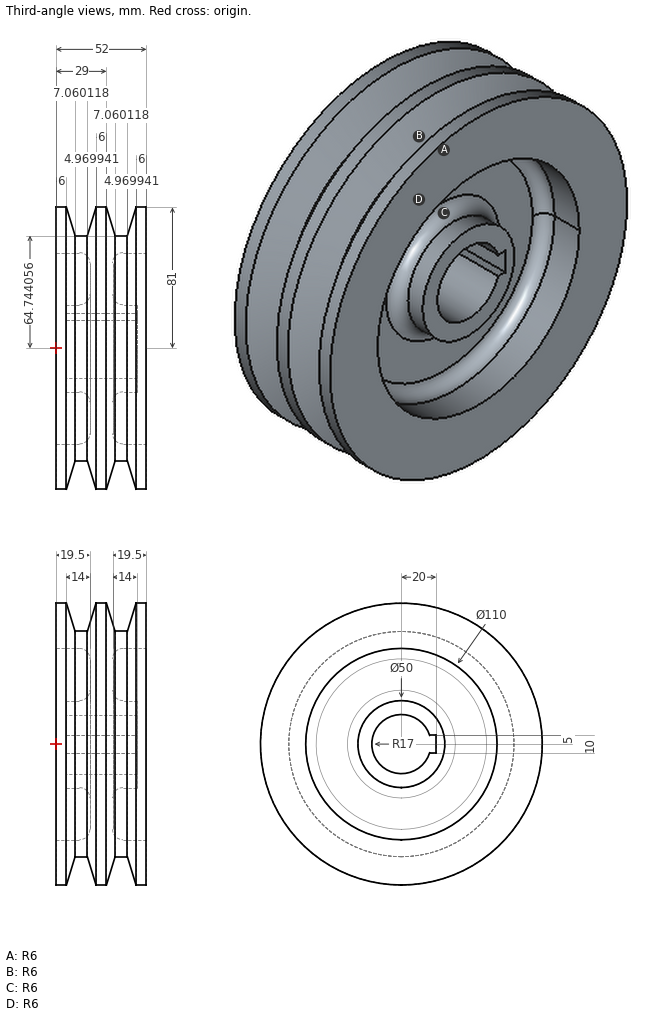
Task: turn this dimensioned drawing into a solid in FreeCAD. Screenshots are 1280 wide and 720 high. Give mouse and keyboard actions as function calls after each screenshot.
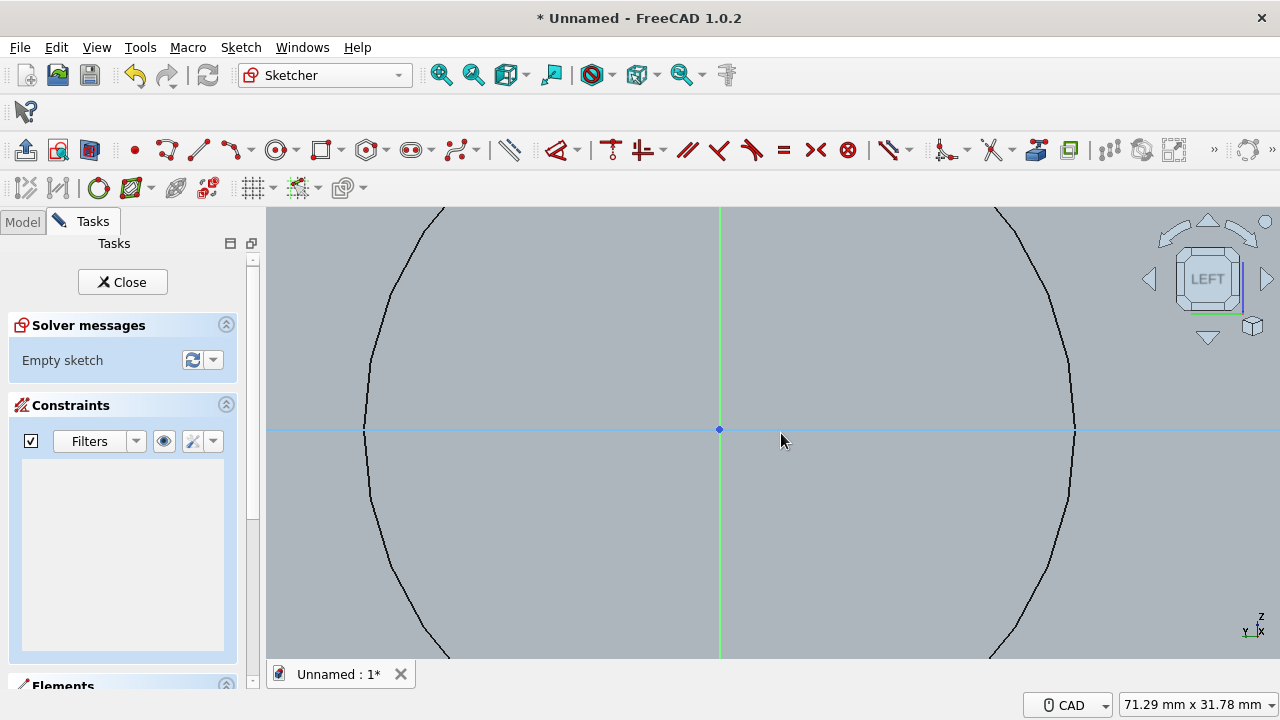
key(g)
key(m)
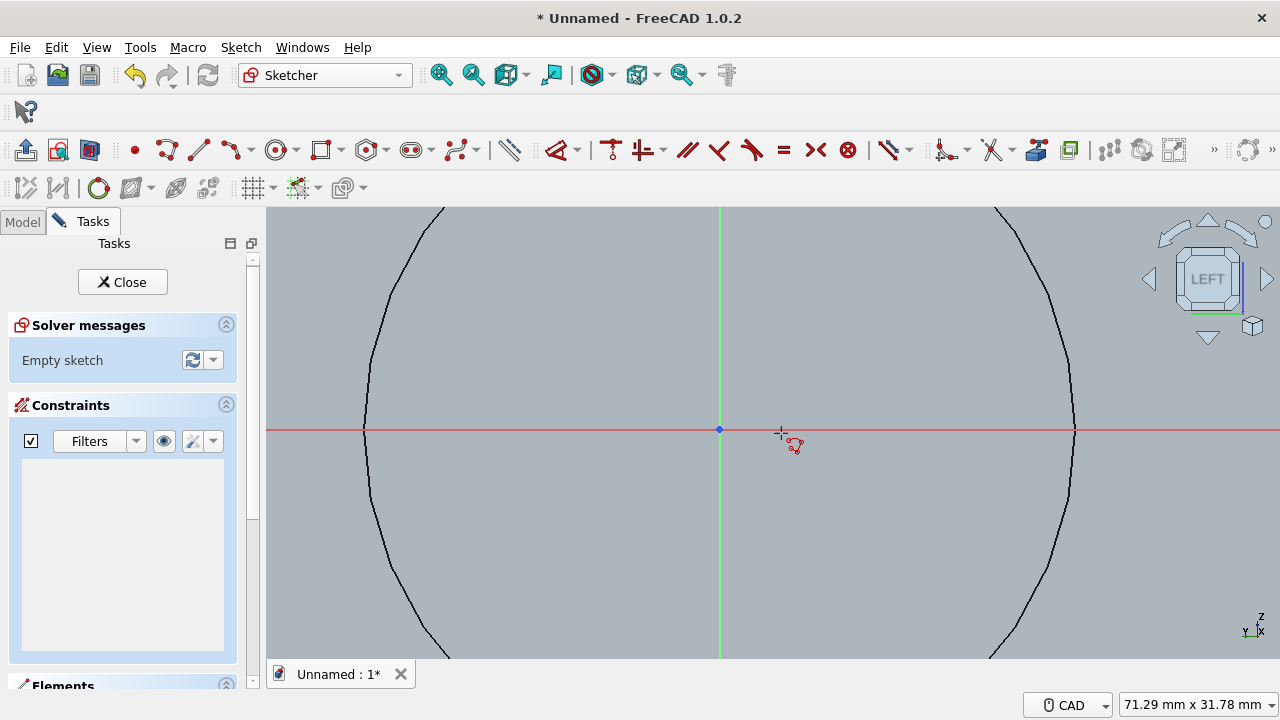
click(488, 359)
click(435, 359)
click(435, 501)
click(488, 501)
right_click(488, 501)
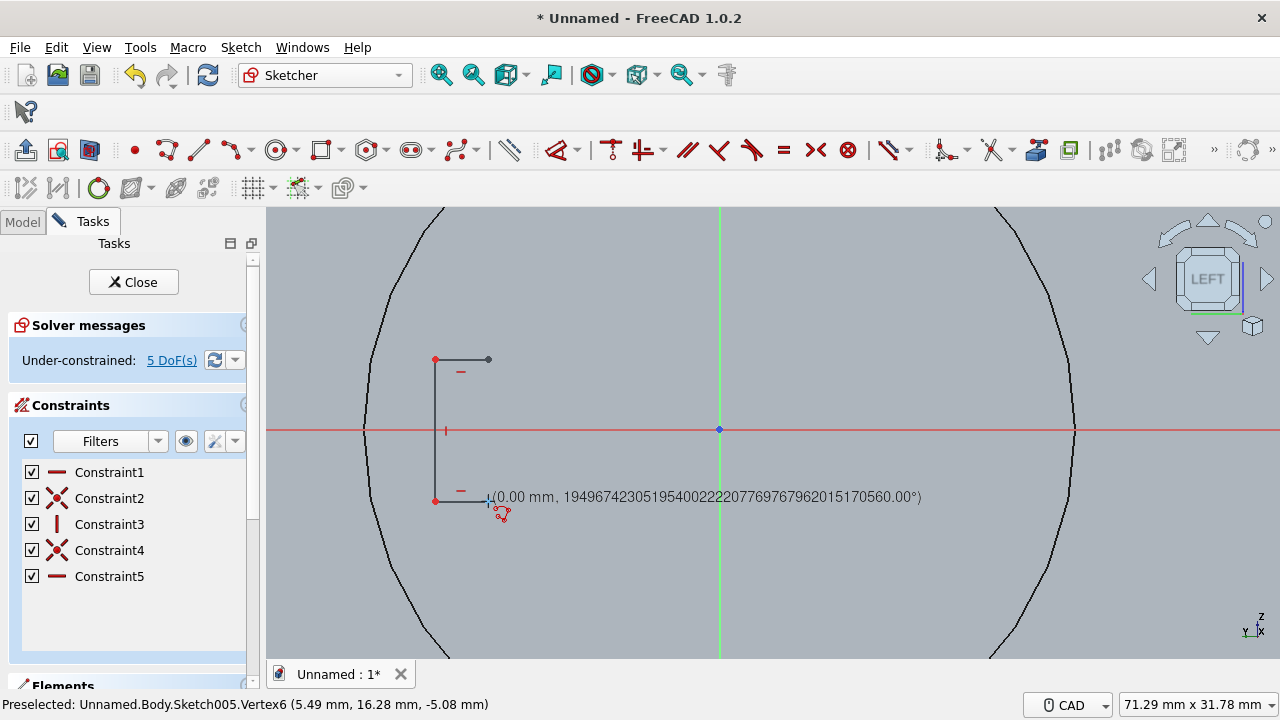
key(g)
key(3)
key(a)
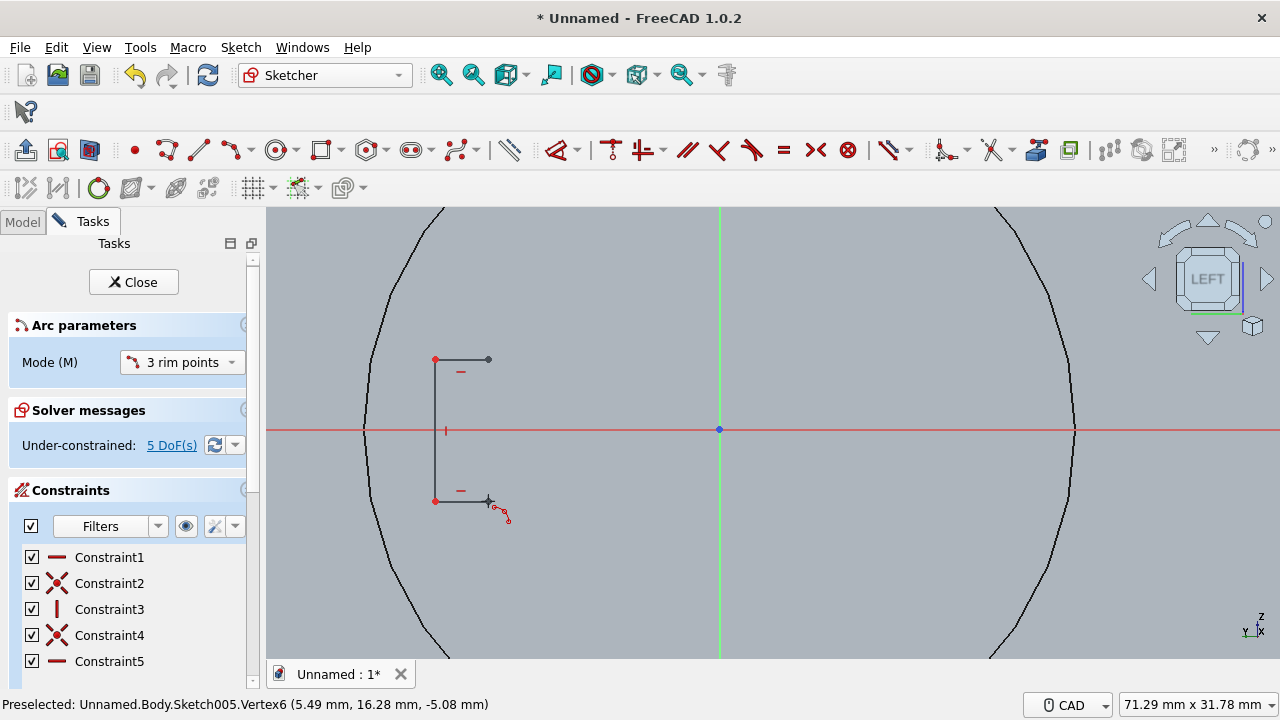
click(488, 502)
click(488, 360)
click(923, 560)
key(Escape)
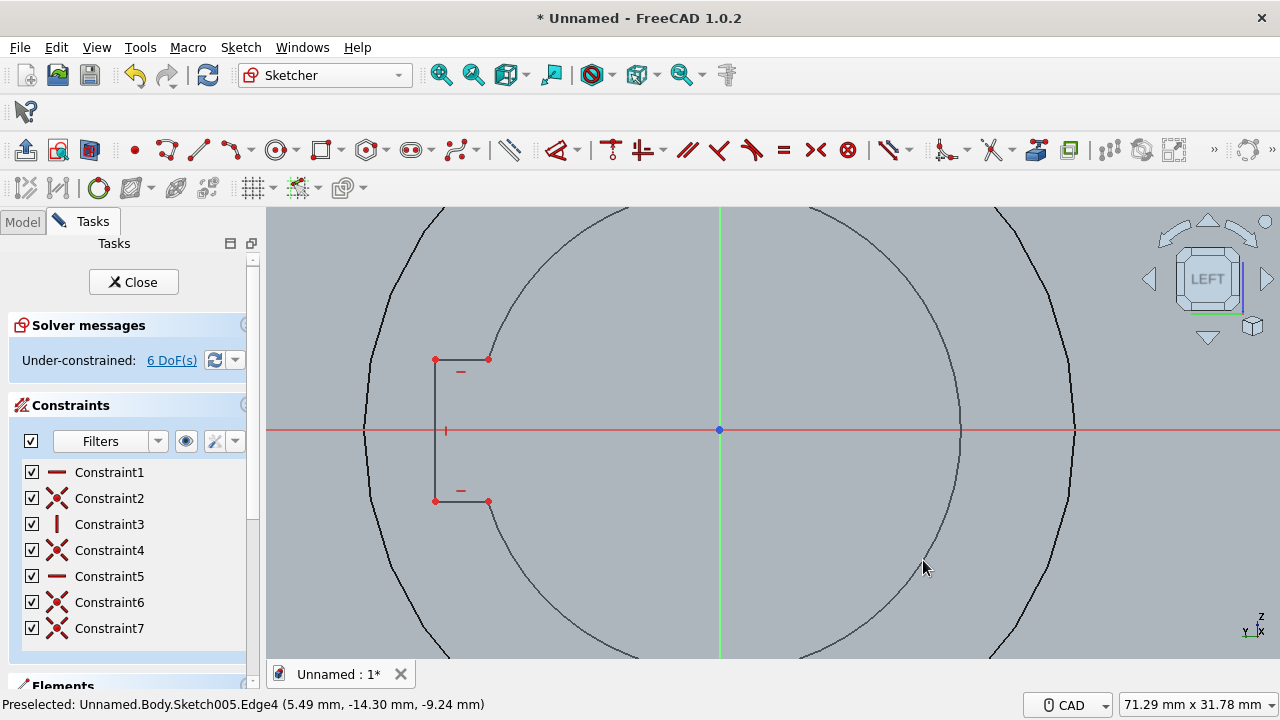
drag(709, 420, 730, 441)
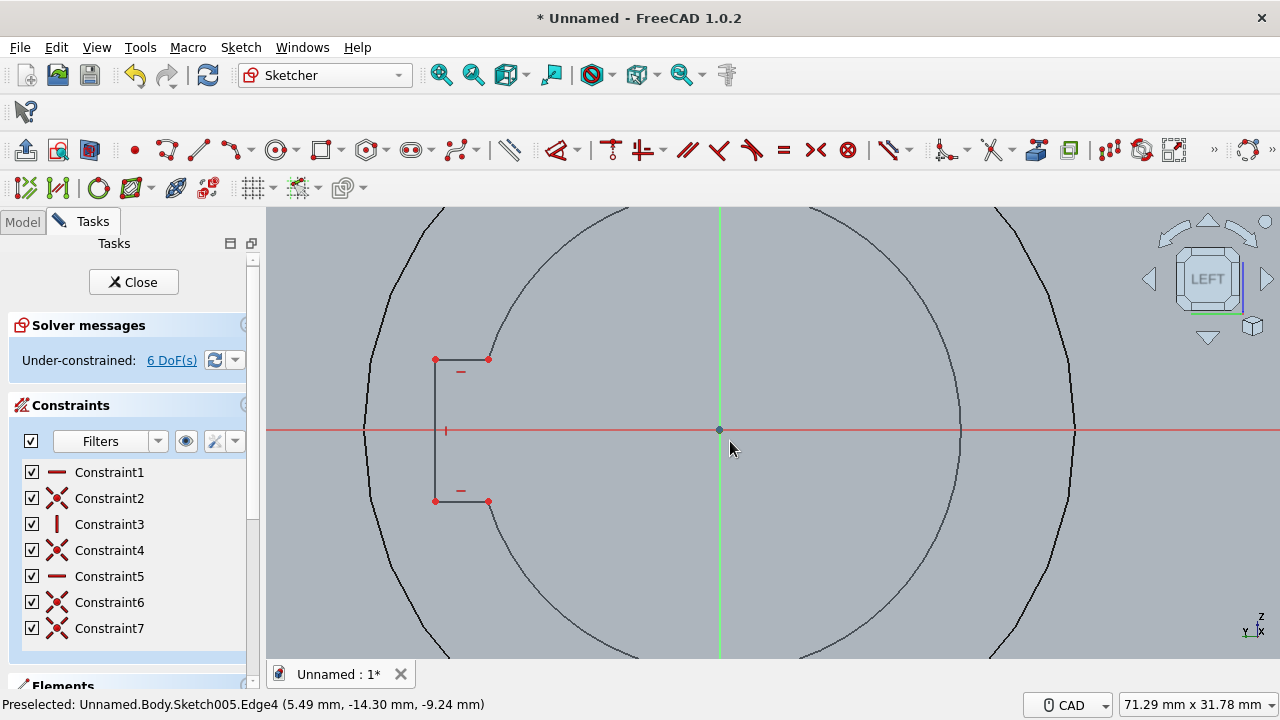
key(c)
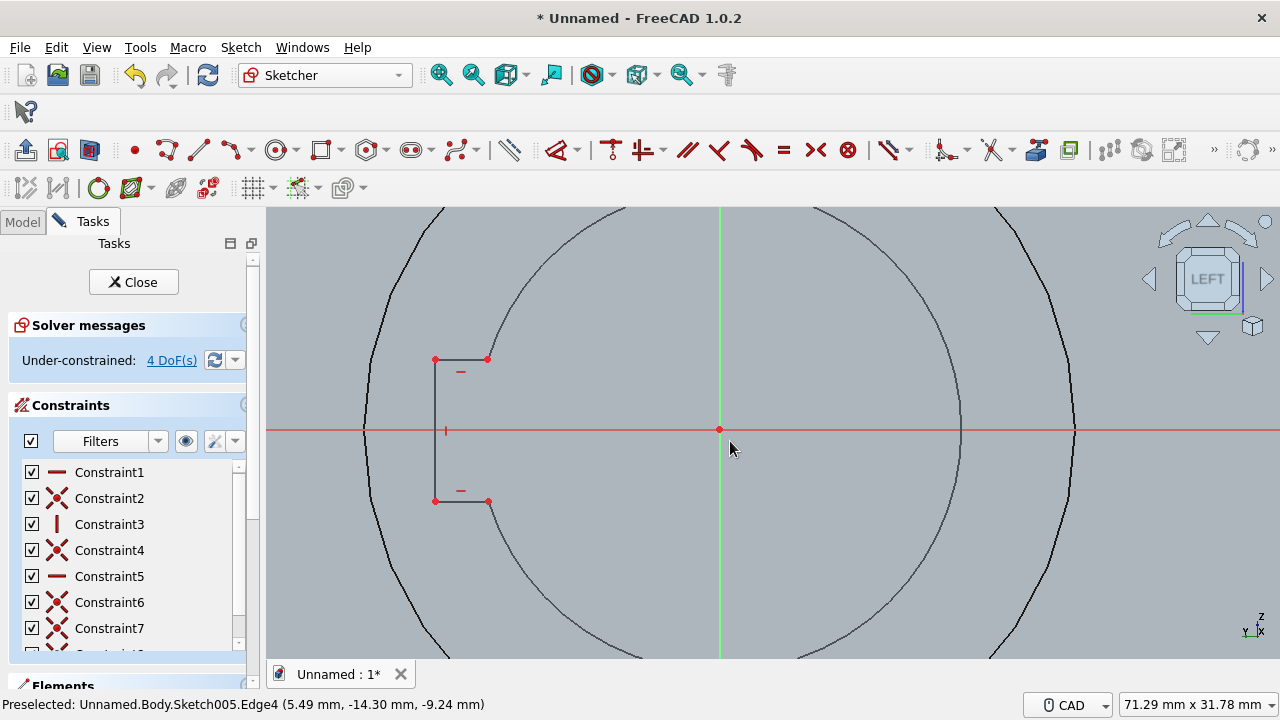
key(d)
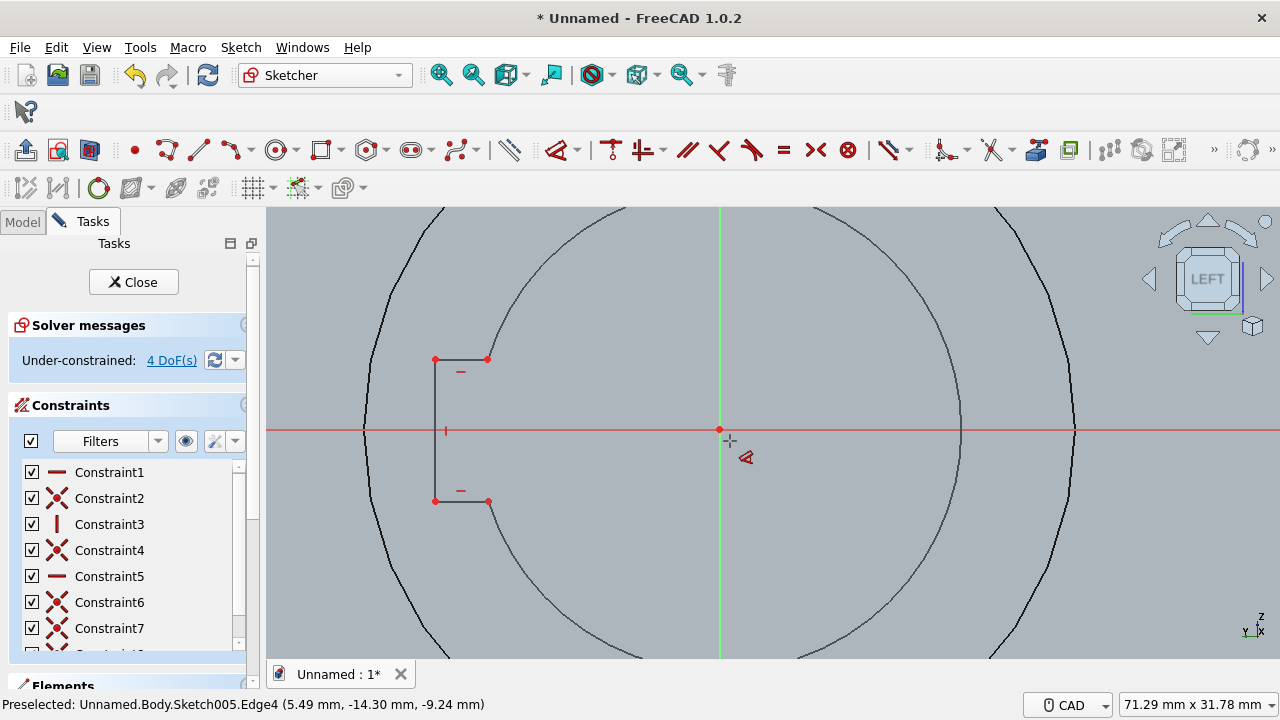
click(961, 429)
click(960, 560)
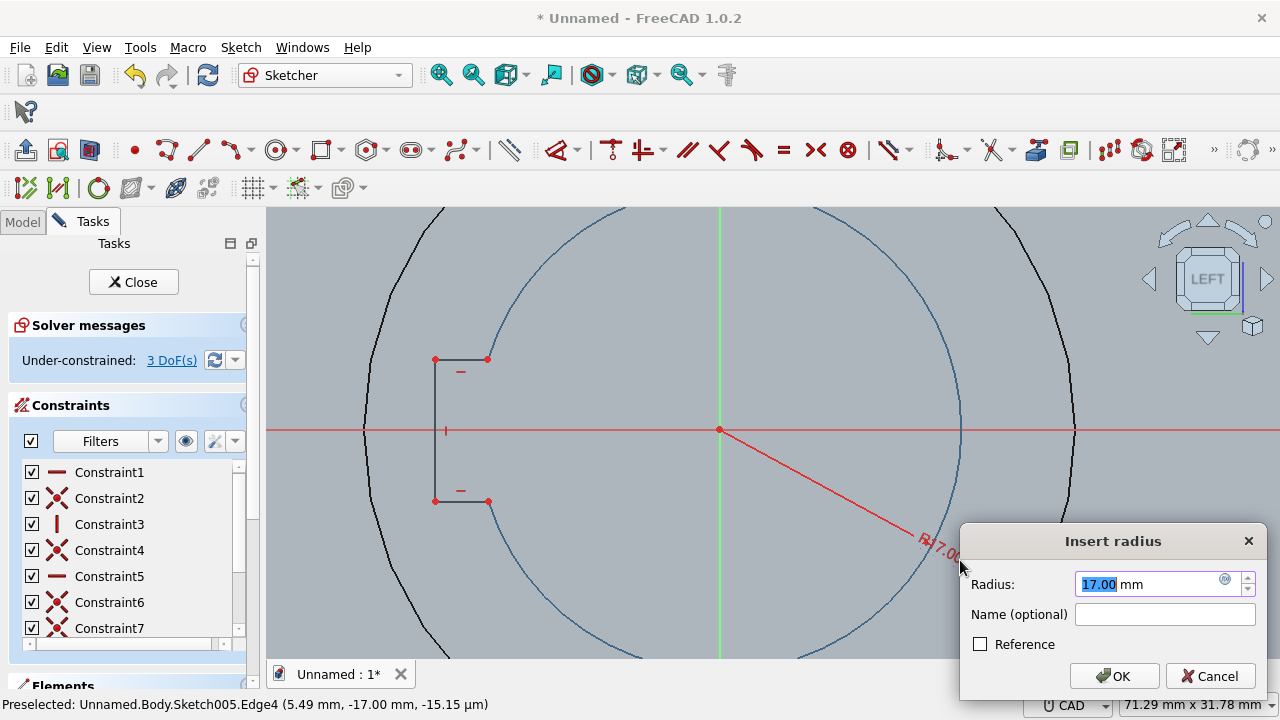
text(17)
key(Return)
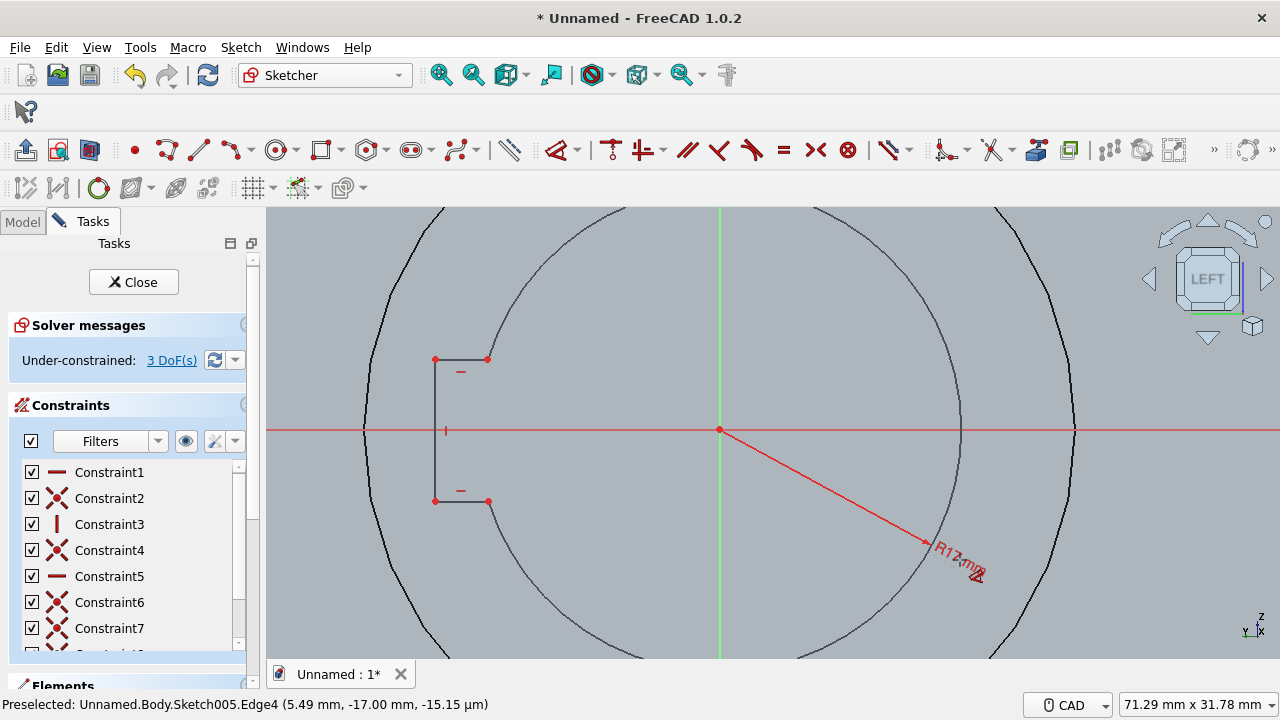
click(435, 403)
click(401, 398)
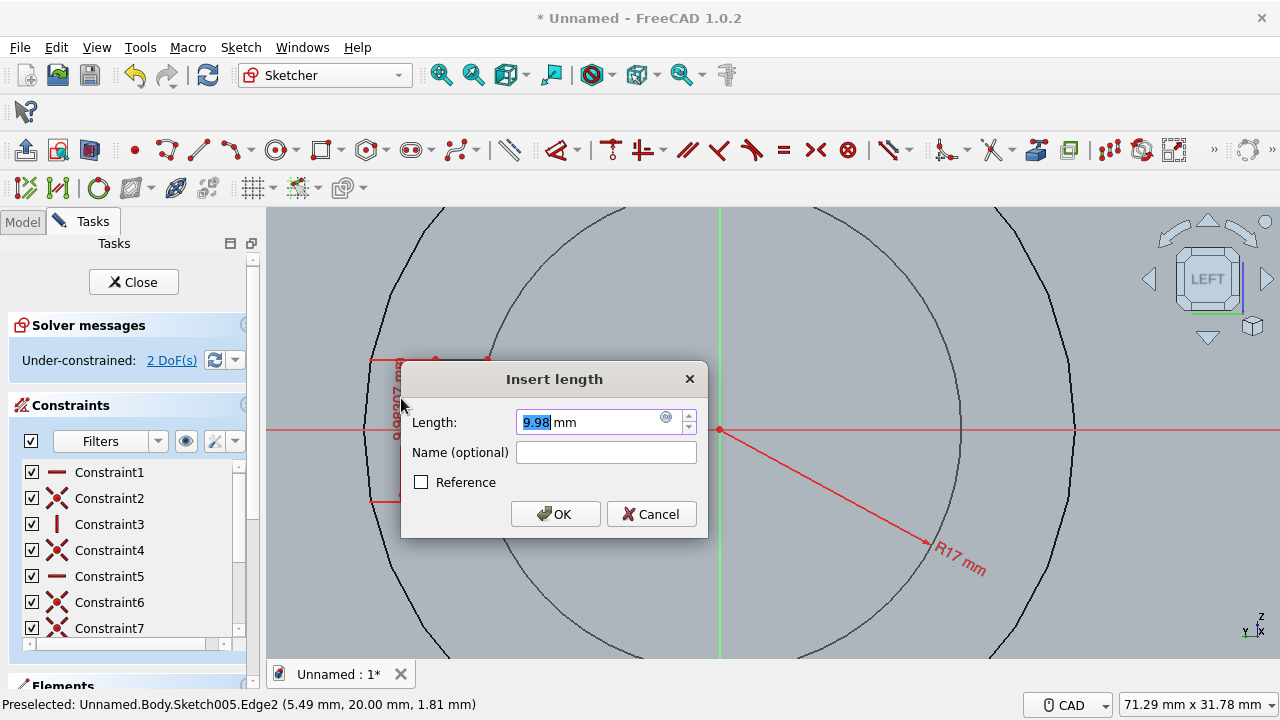
text(10)
key(Return)